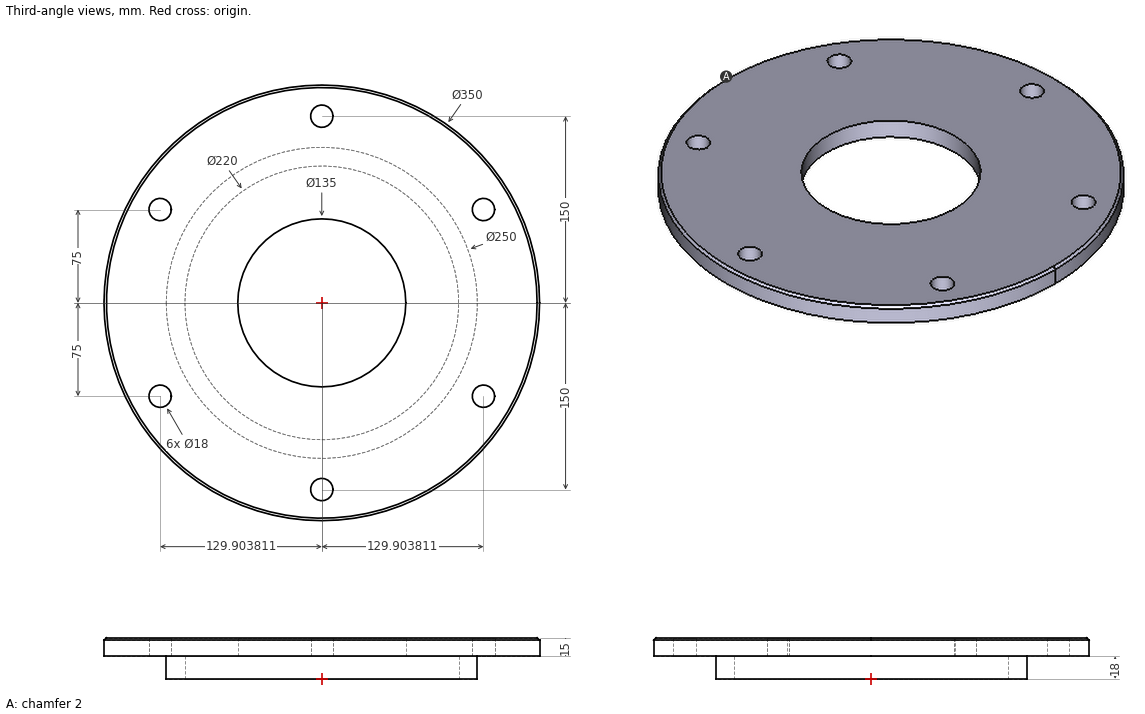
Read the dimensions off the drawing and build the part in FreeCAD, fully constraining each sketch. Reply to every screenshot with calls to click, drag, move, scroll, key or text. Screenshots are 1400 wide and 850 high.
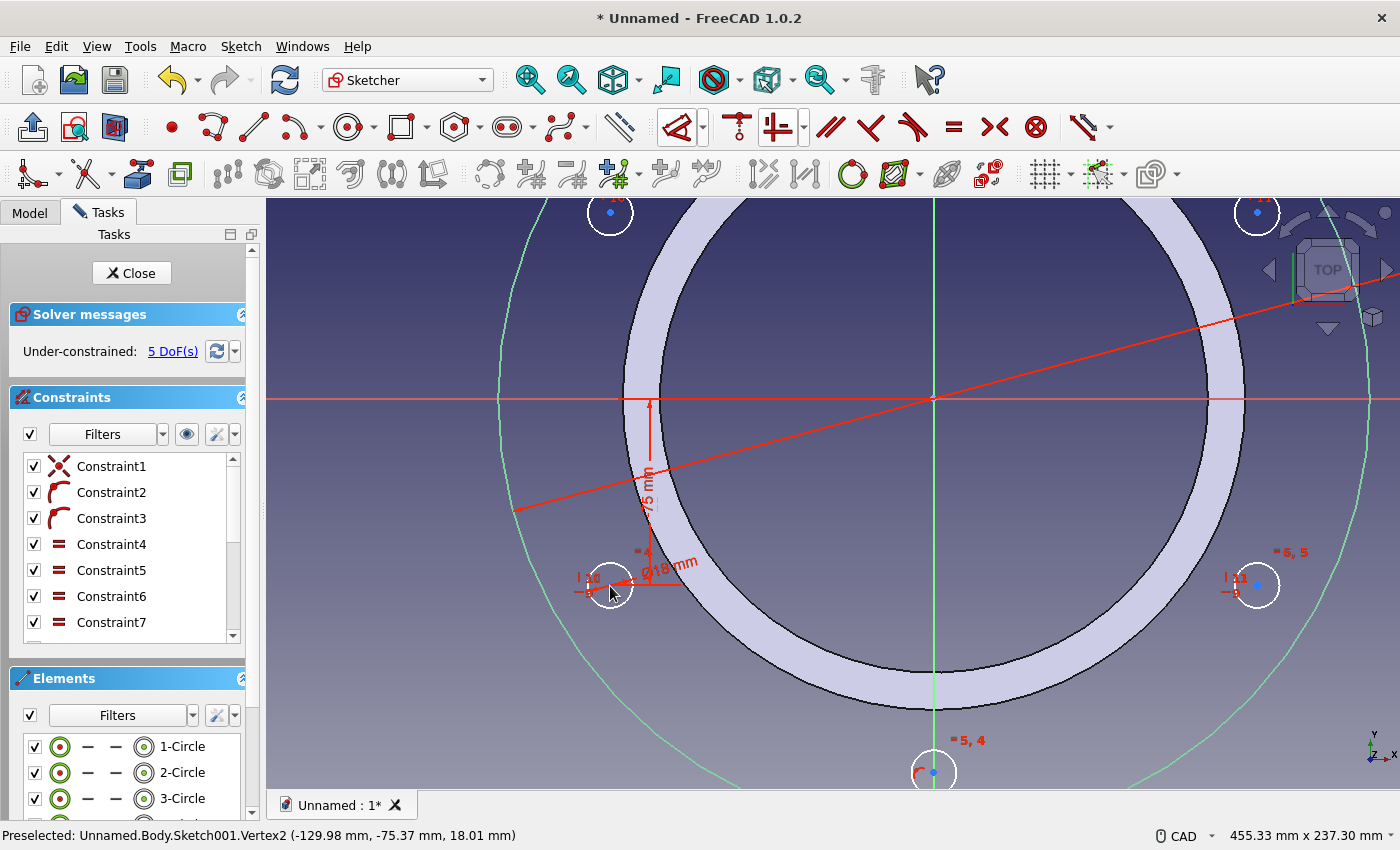
scroll(626, 571, down, 4)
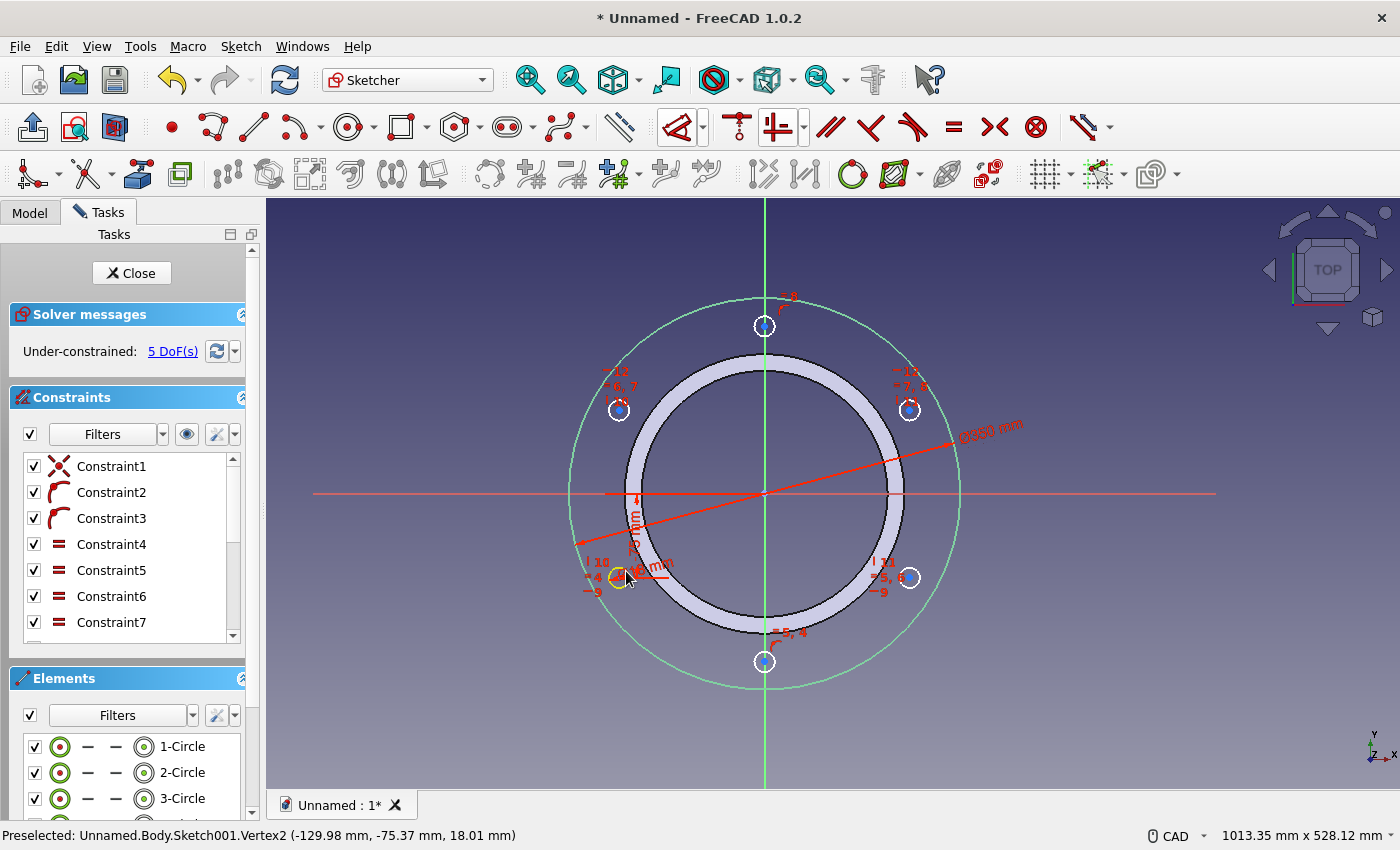
click(619, 410)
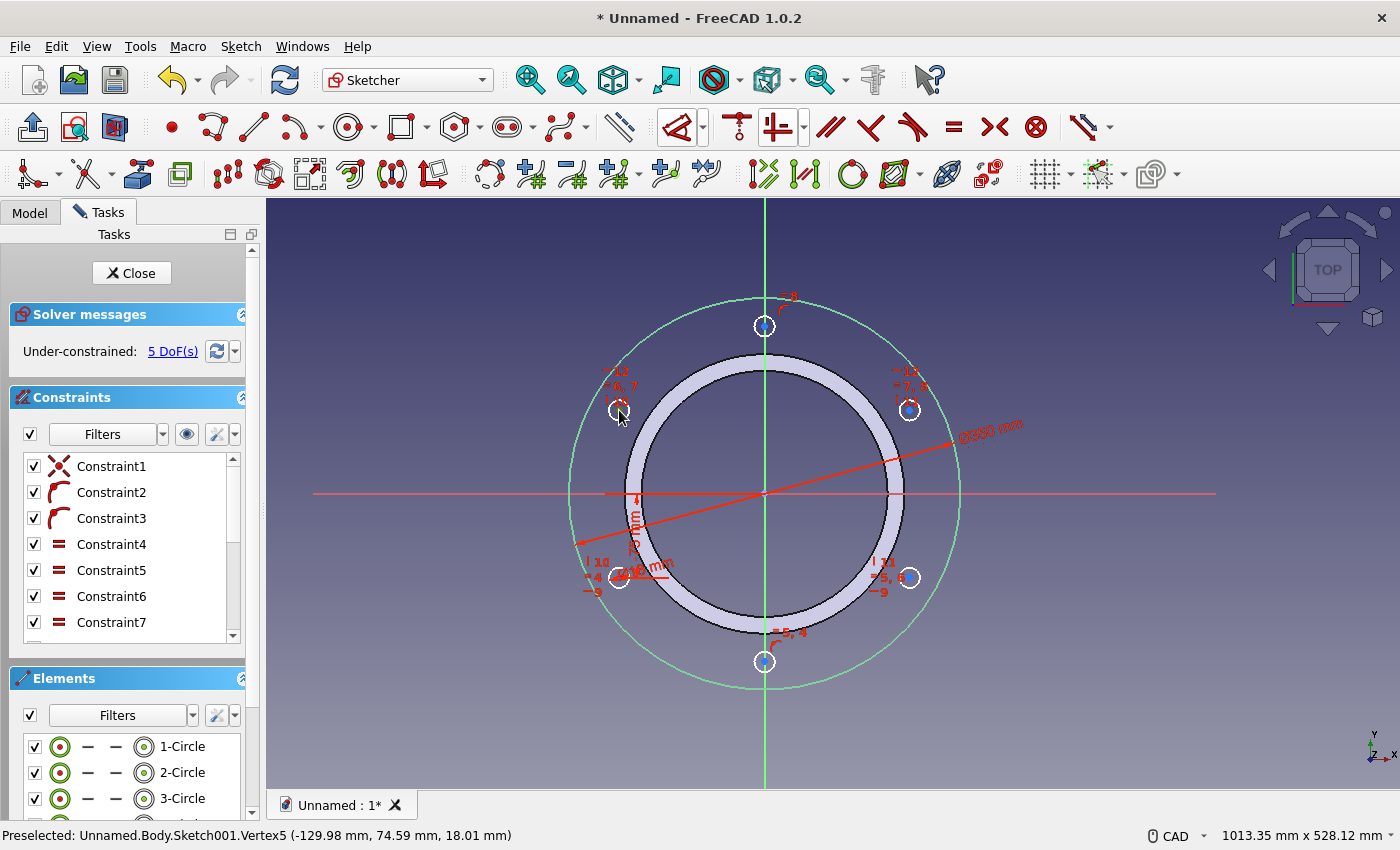
key(i)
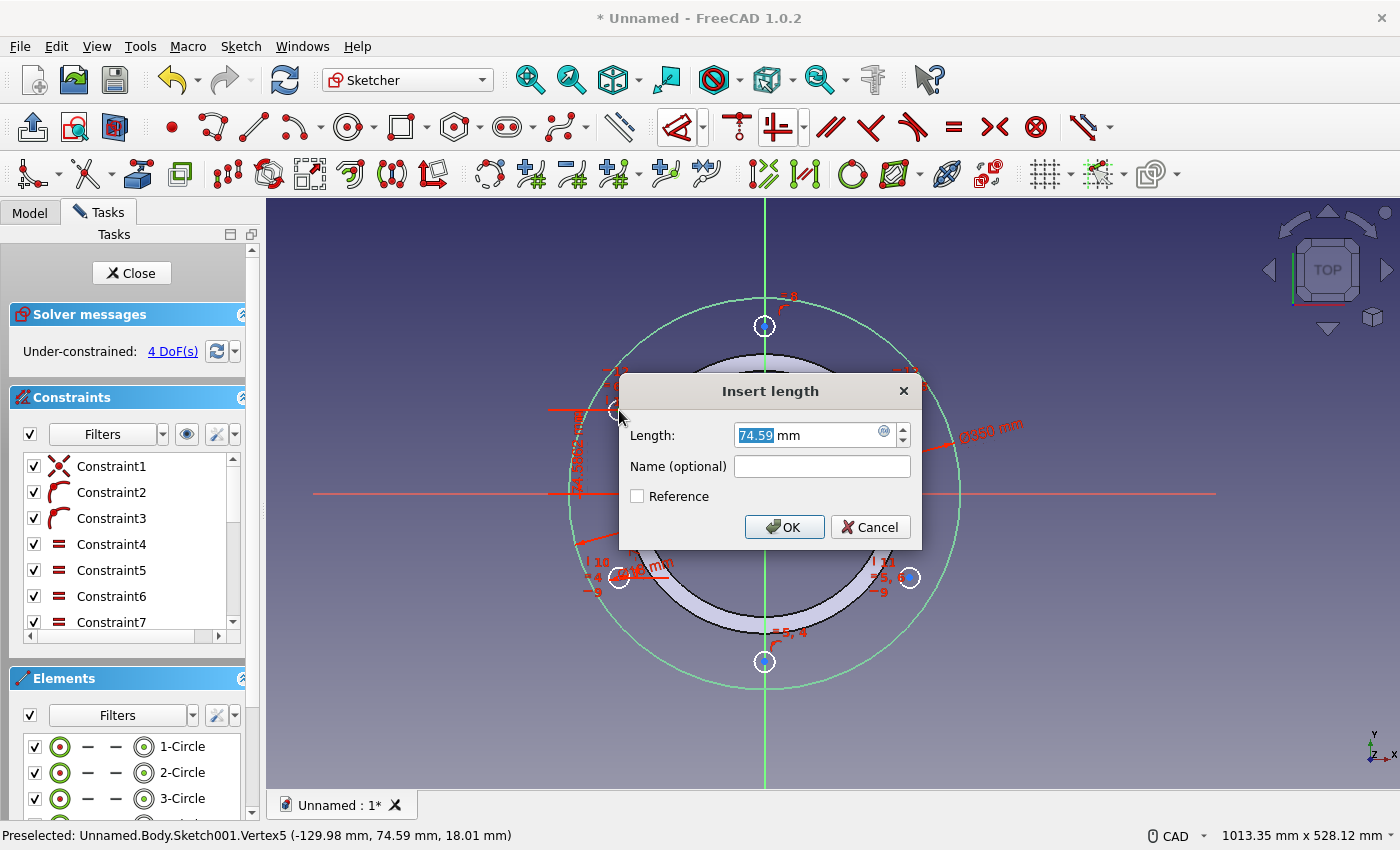
text(75)
key(Return)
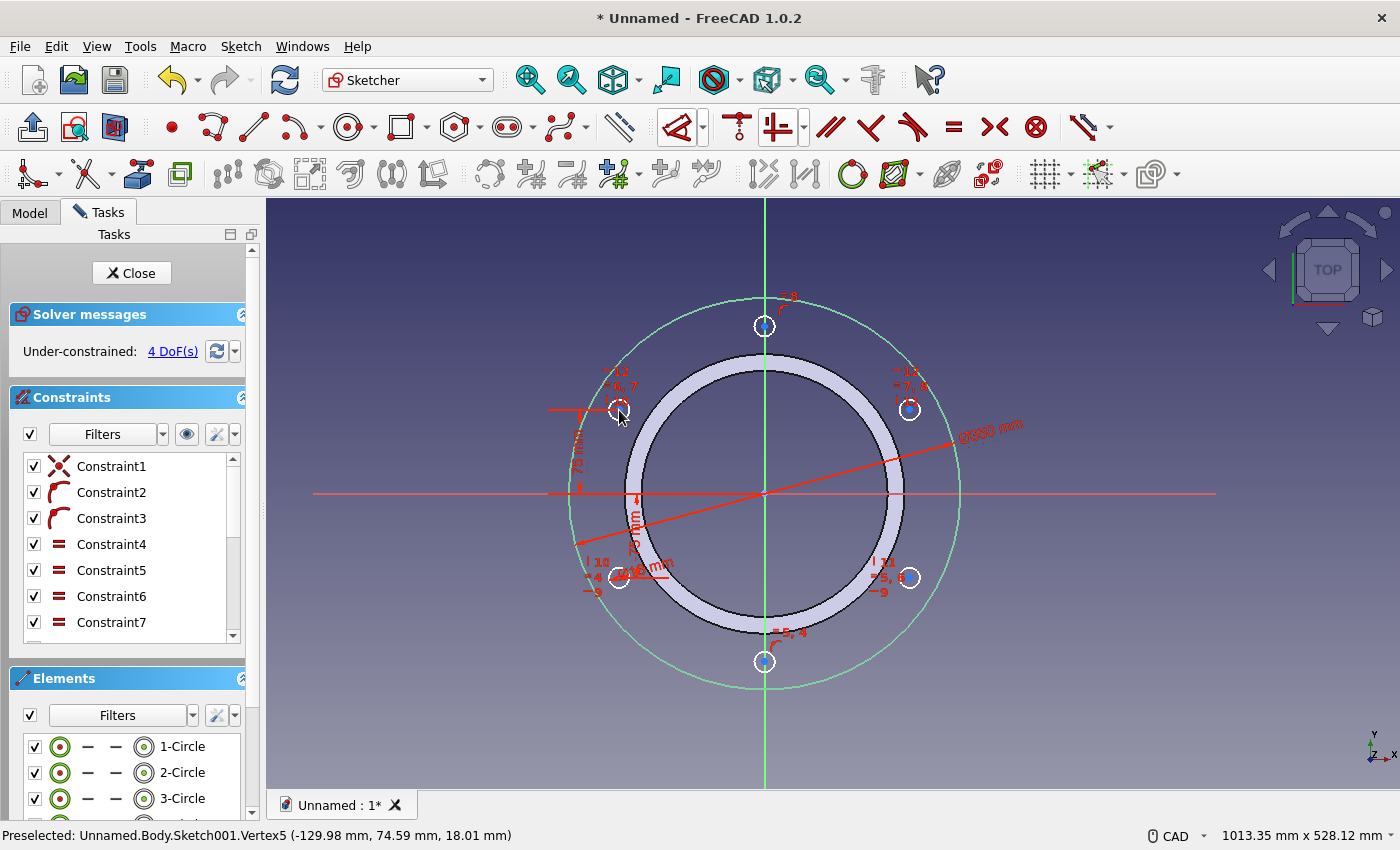
click(765, 662)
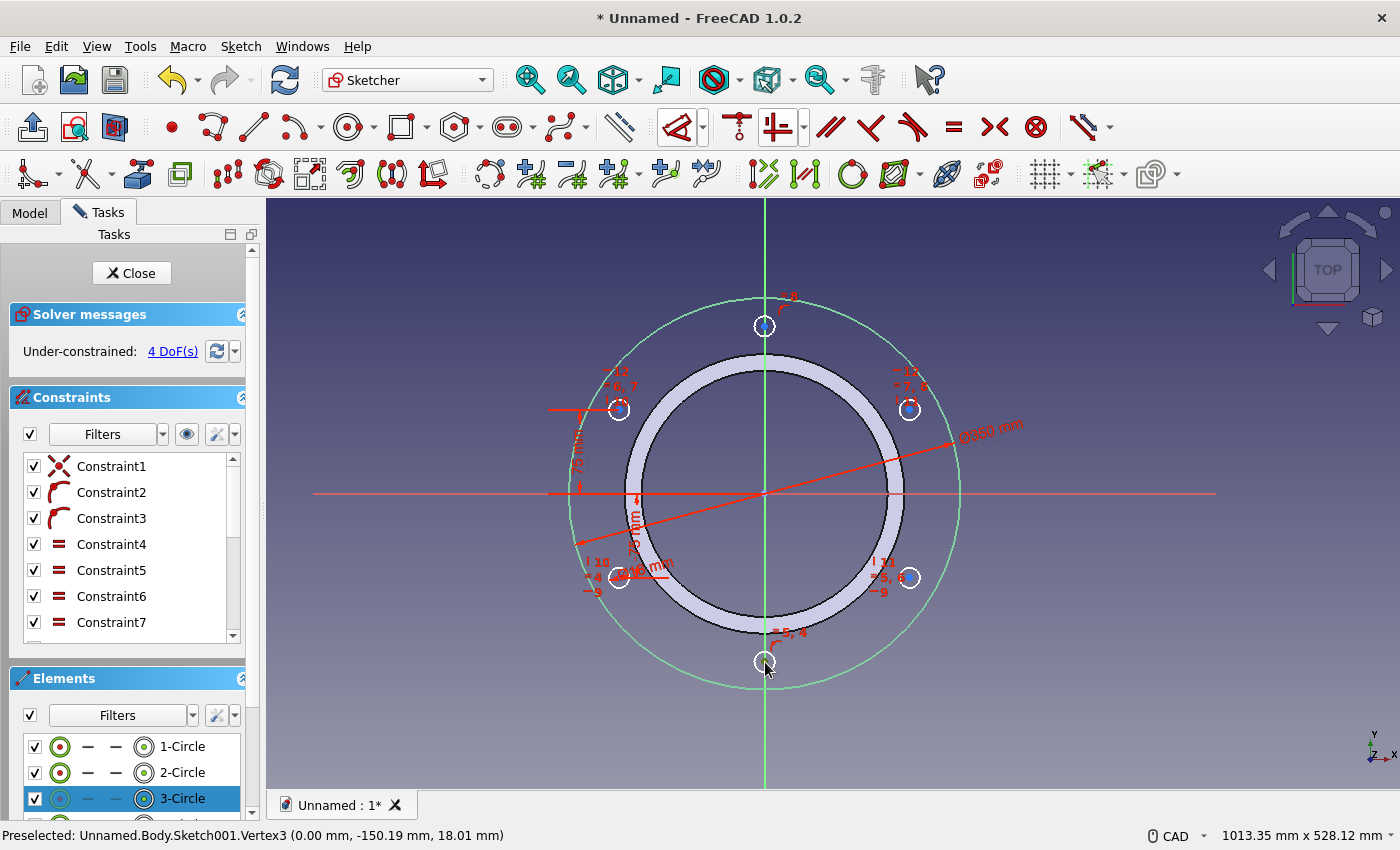
key(i)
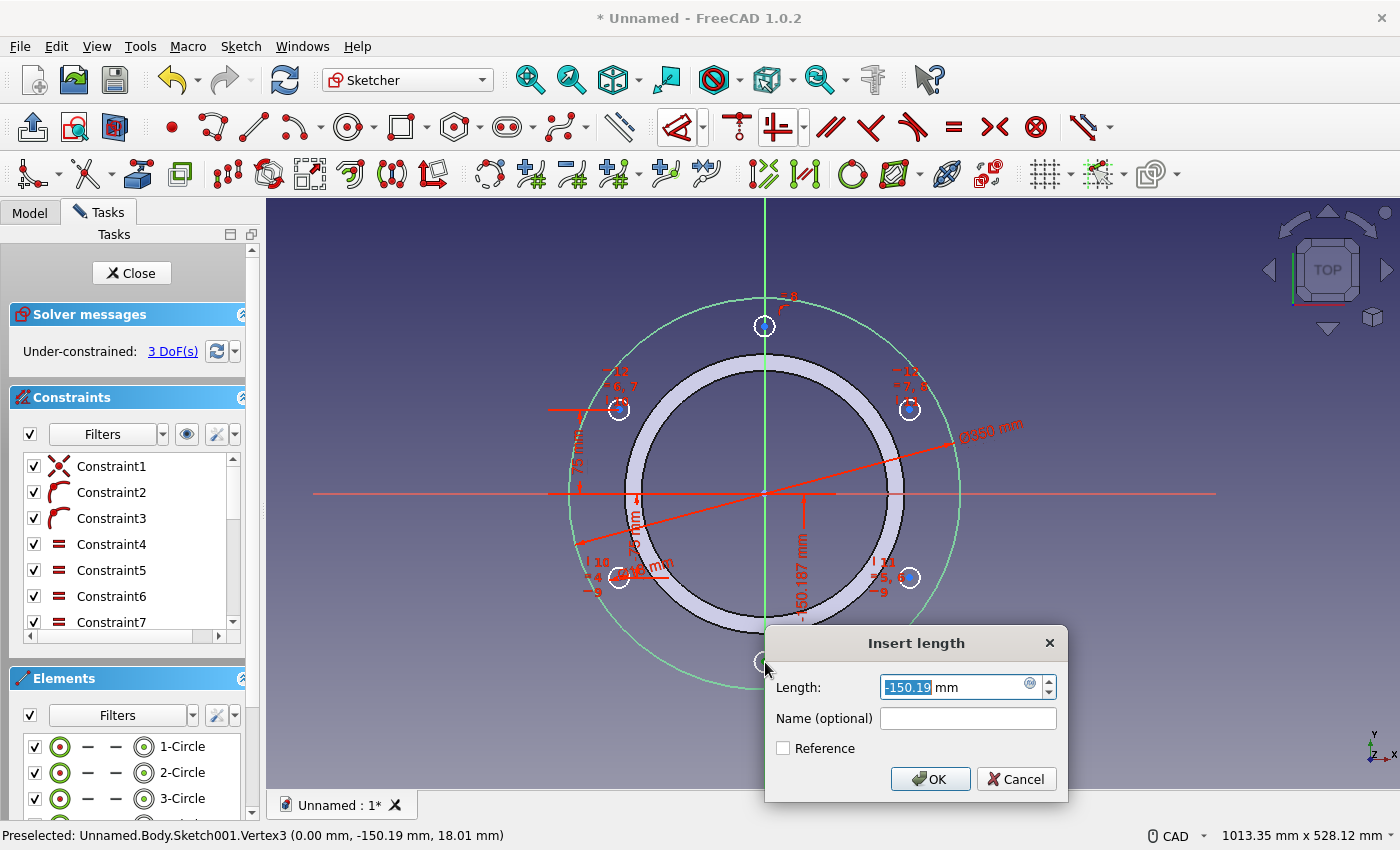
text(-150)
key(Return)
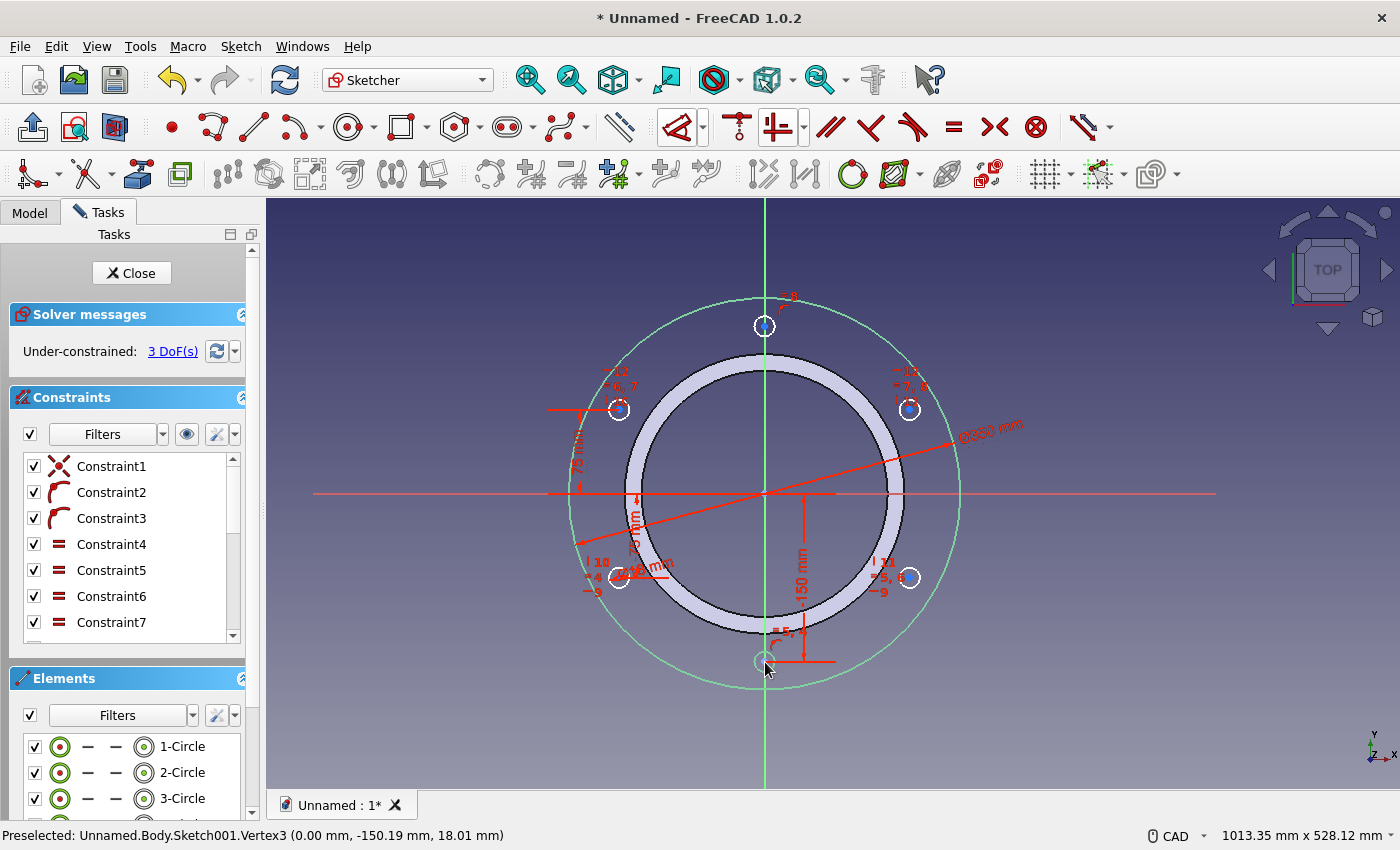
click(765, 326)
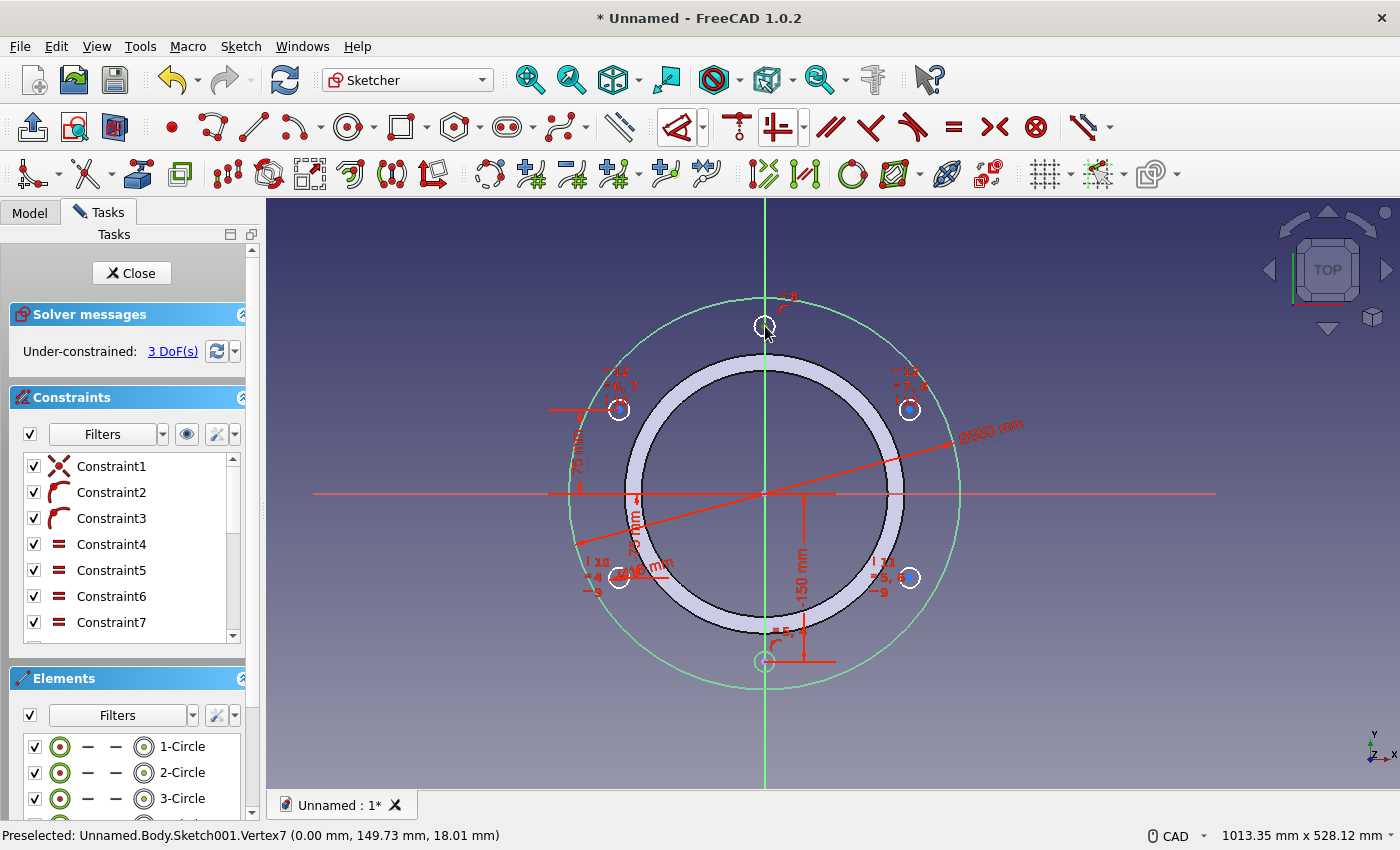
key(i)